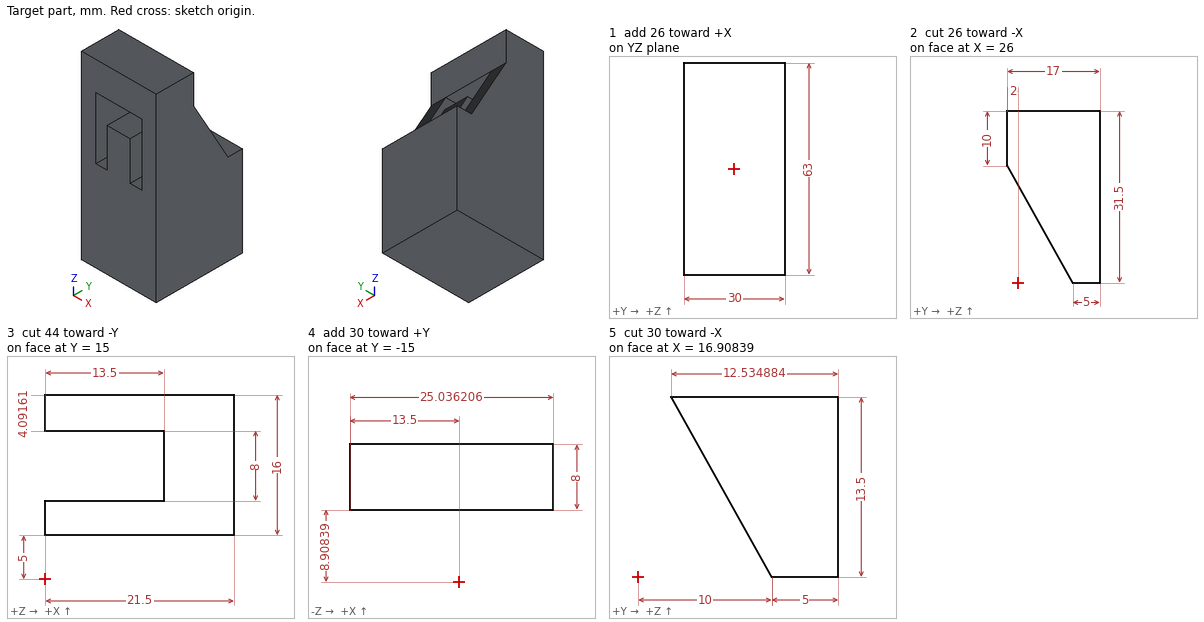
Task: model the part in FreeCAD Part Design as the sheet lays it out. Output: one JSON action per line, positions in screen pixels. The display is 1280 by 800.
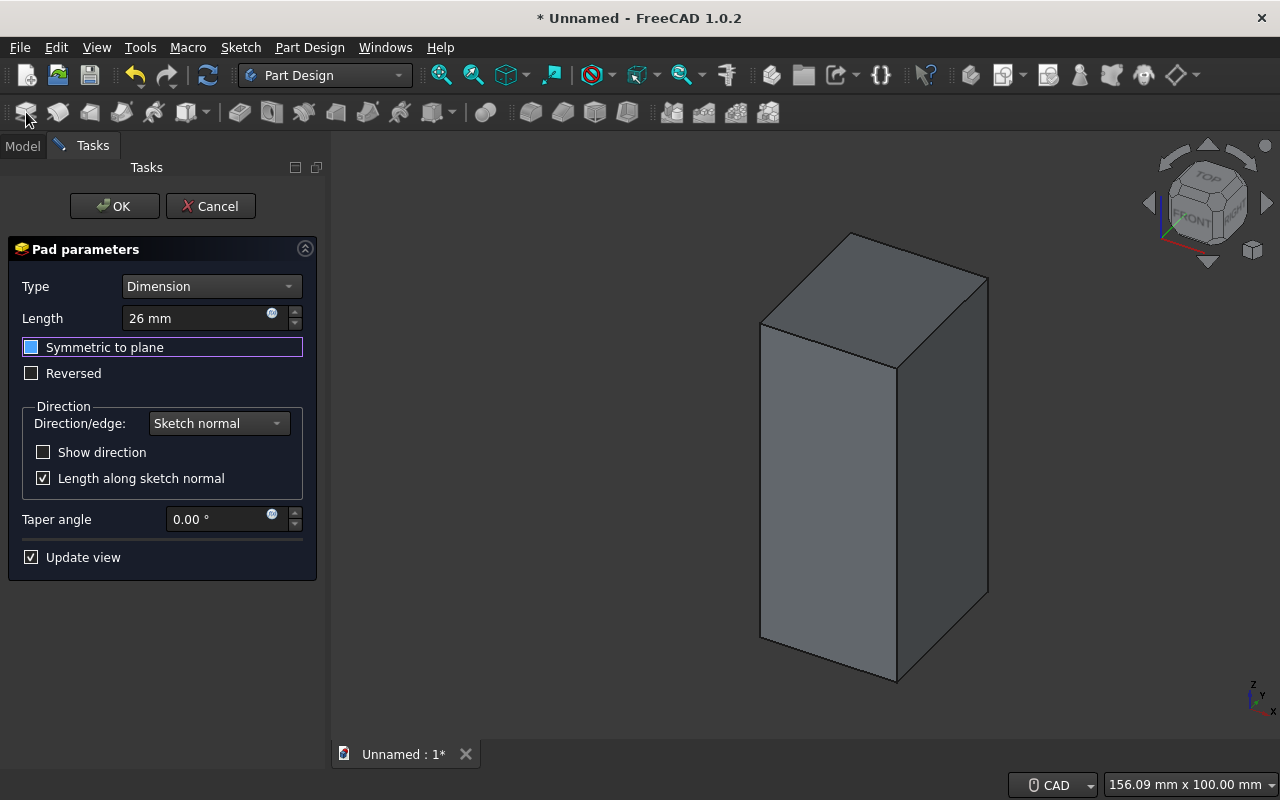
{"action": "left_click", "coordinate": [115, 206]}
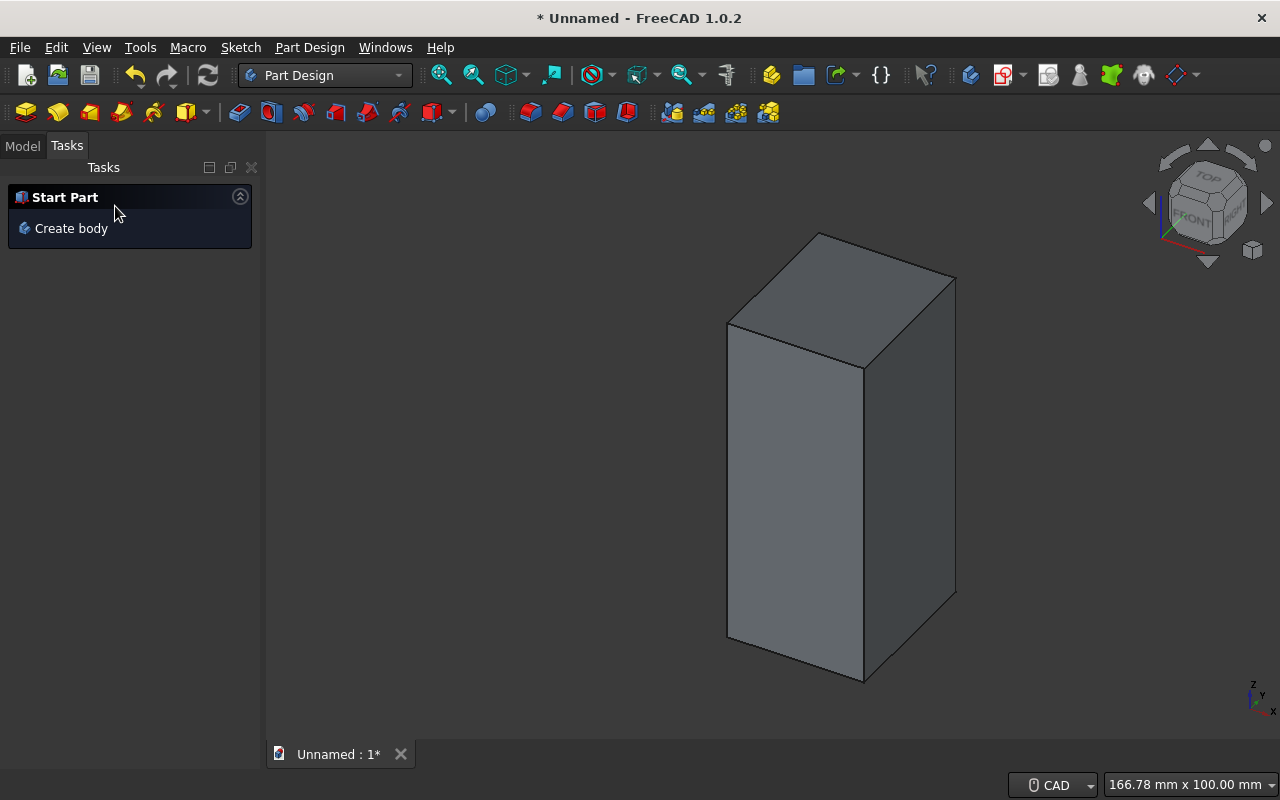
{"action": "left_click", "coordinate": [910, 524]}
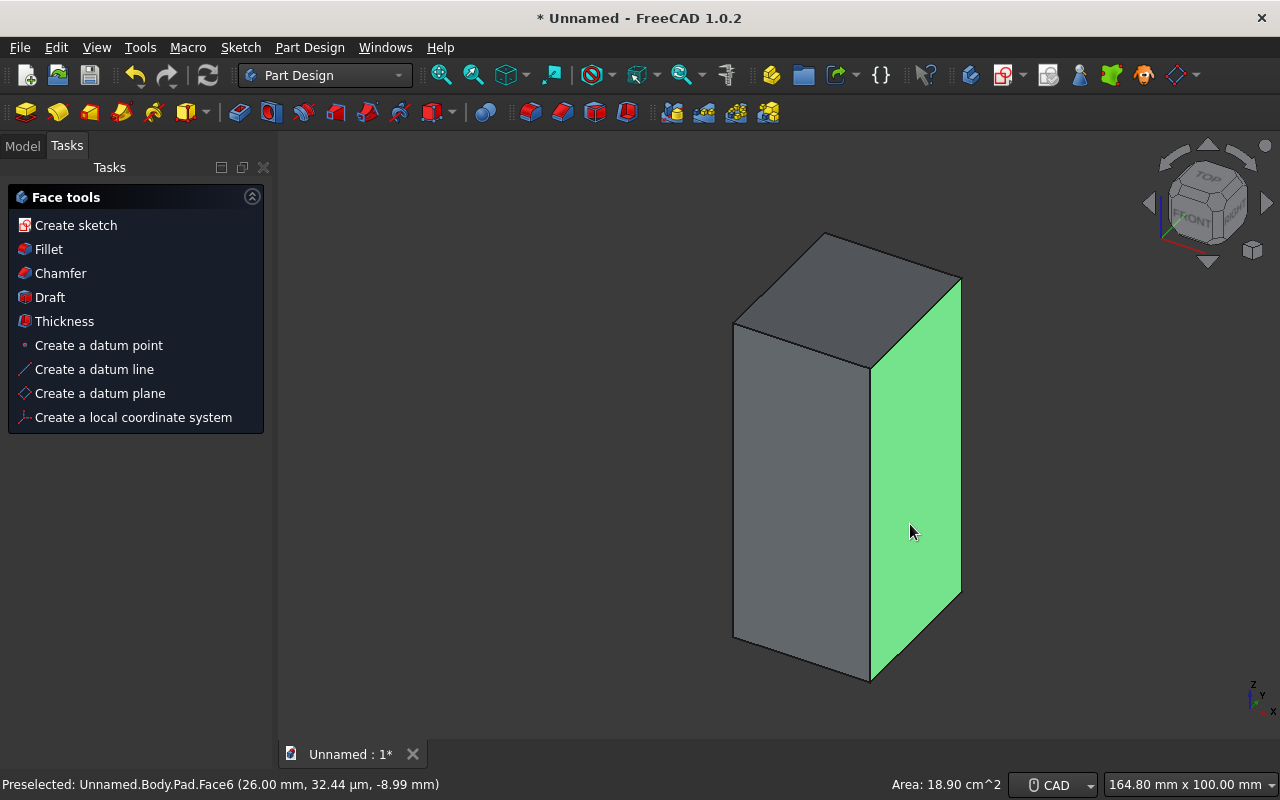
{"action": "left_click", "coordinate": [1004, 76]}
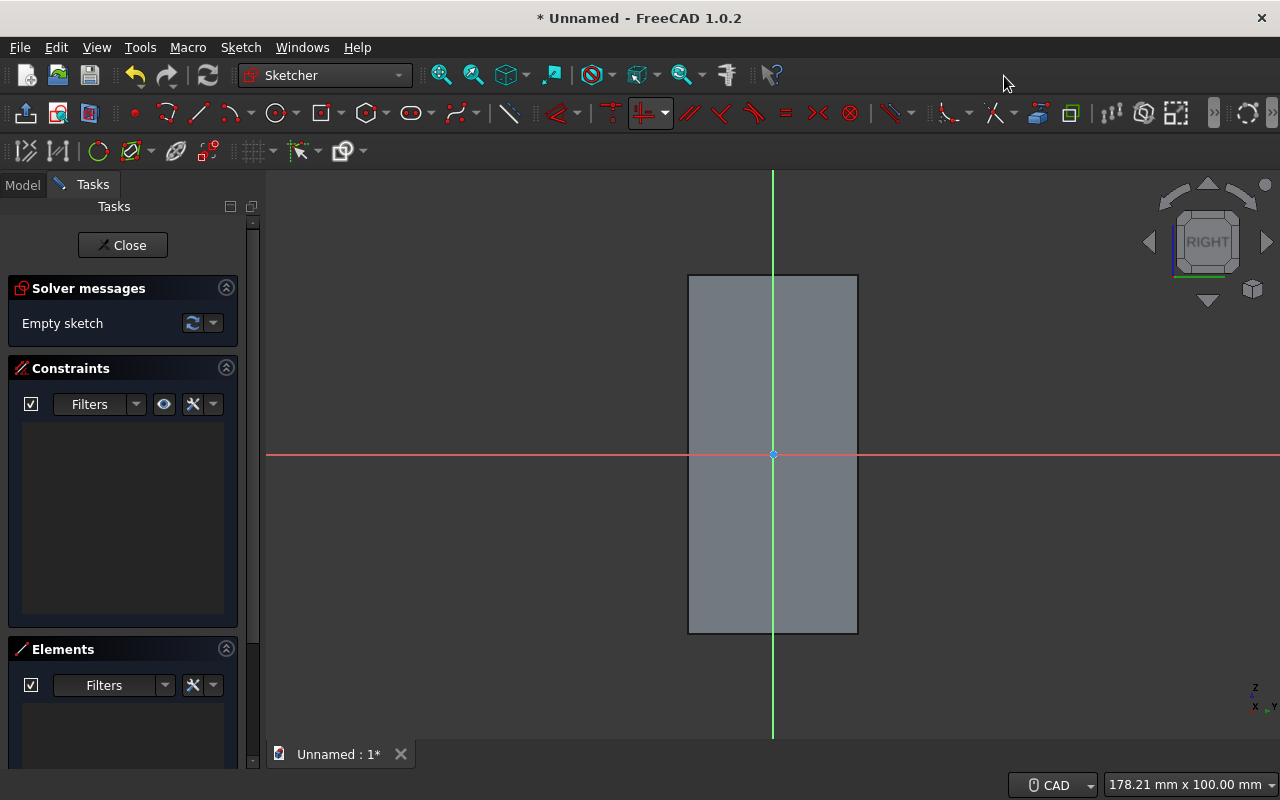
{"action": "scroll", "coordinate": [896, 292], "scroll_direction": "up", "scroll_amount": 4}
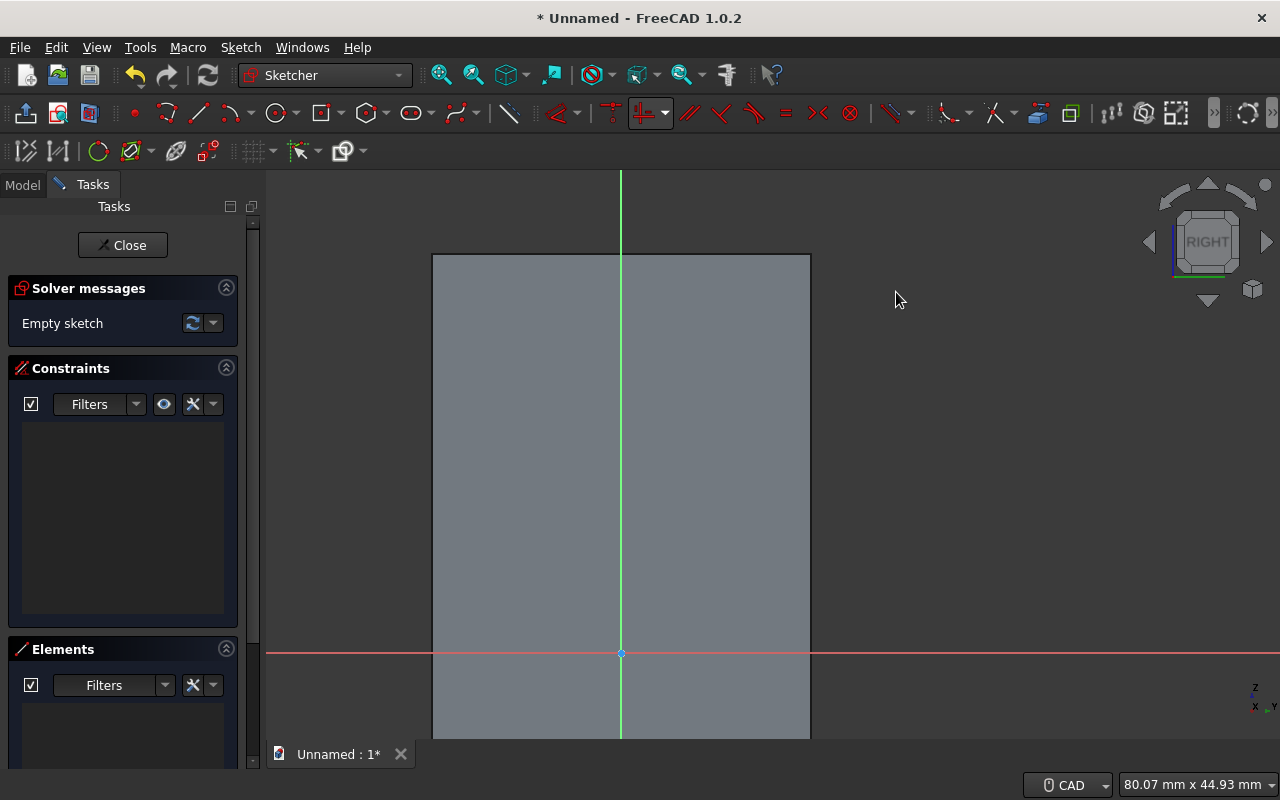
{"action": "key", "text": "g m"}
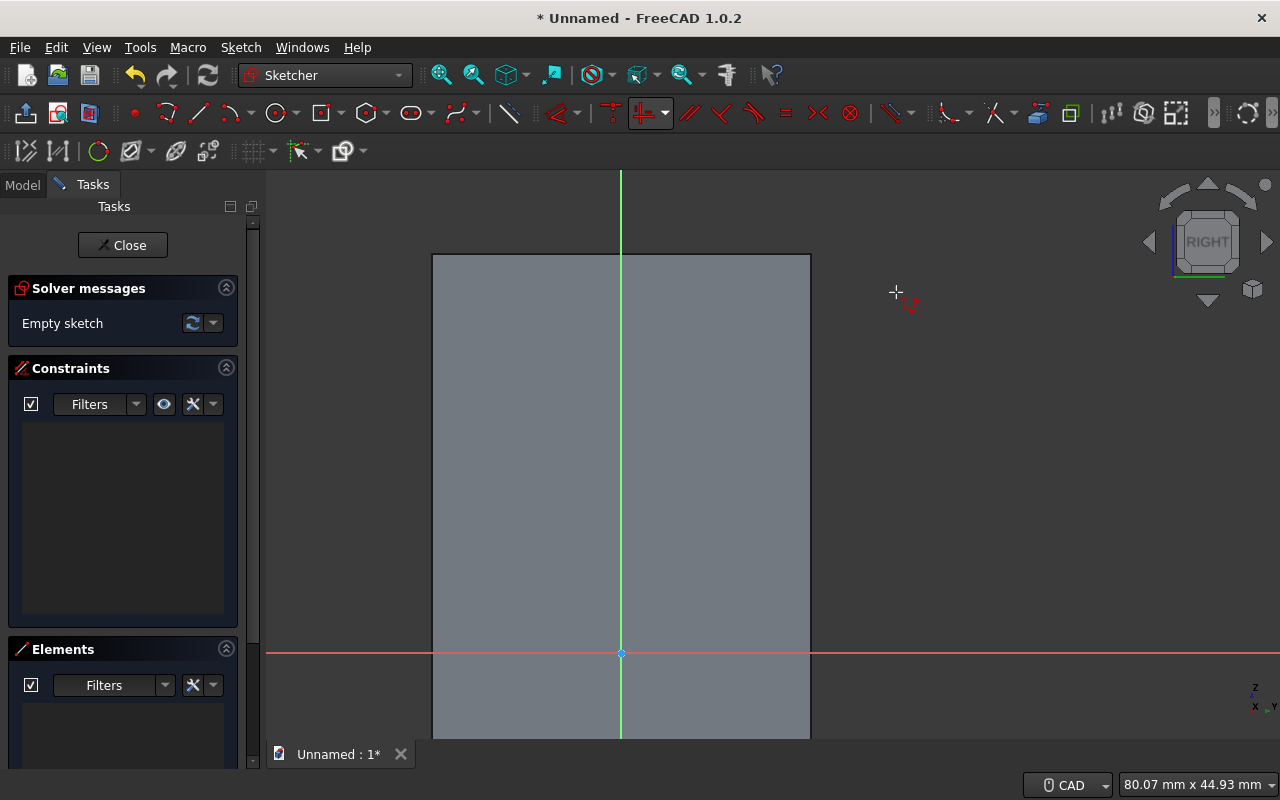
{"action": "left_click", "coordinate": [748, 653]}
{"action": "left_click", "coordinate": [811, 644]}
{"action": "left_click", "coordinate": [811, 254]}
{"action": "left_click", "coordinate": [596, 254]}
{"action": "left_click", "coordinate": [596, 381]}
{"action": "left_click", "coordinate": [748, 653]}
{"action": "key", "text": "Escape"}
{"action": "key", "text": "Escape"}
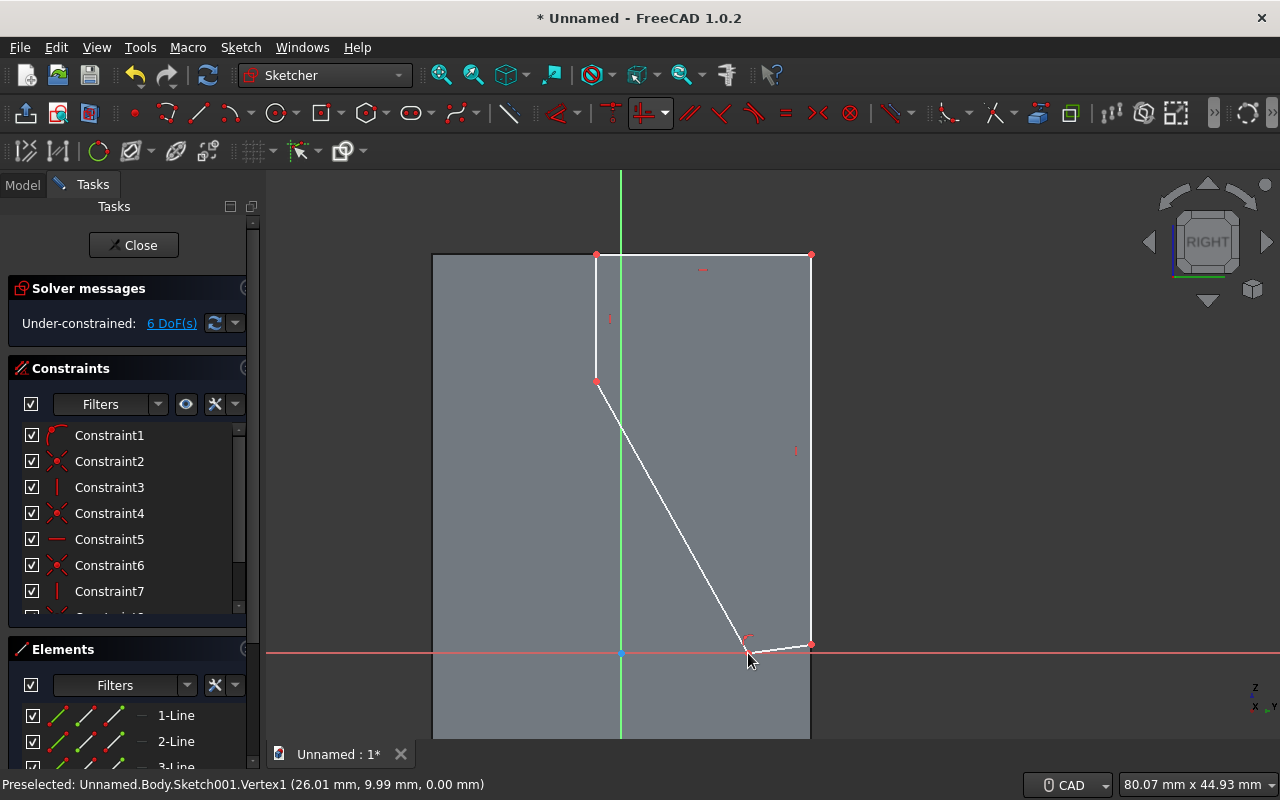
{"action": "left_click", "coordinate": [767, 651]}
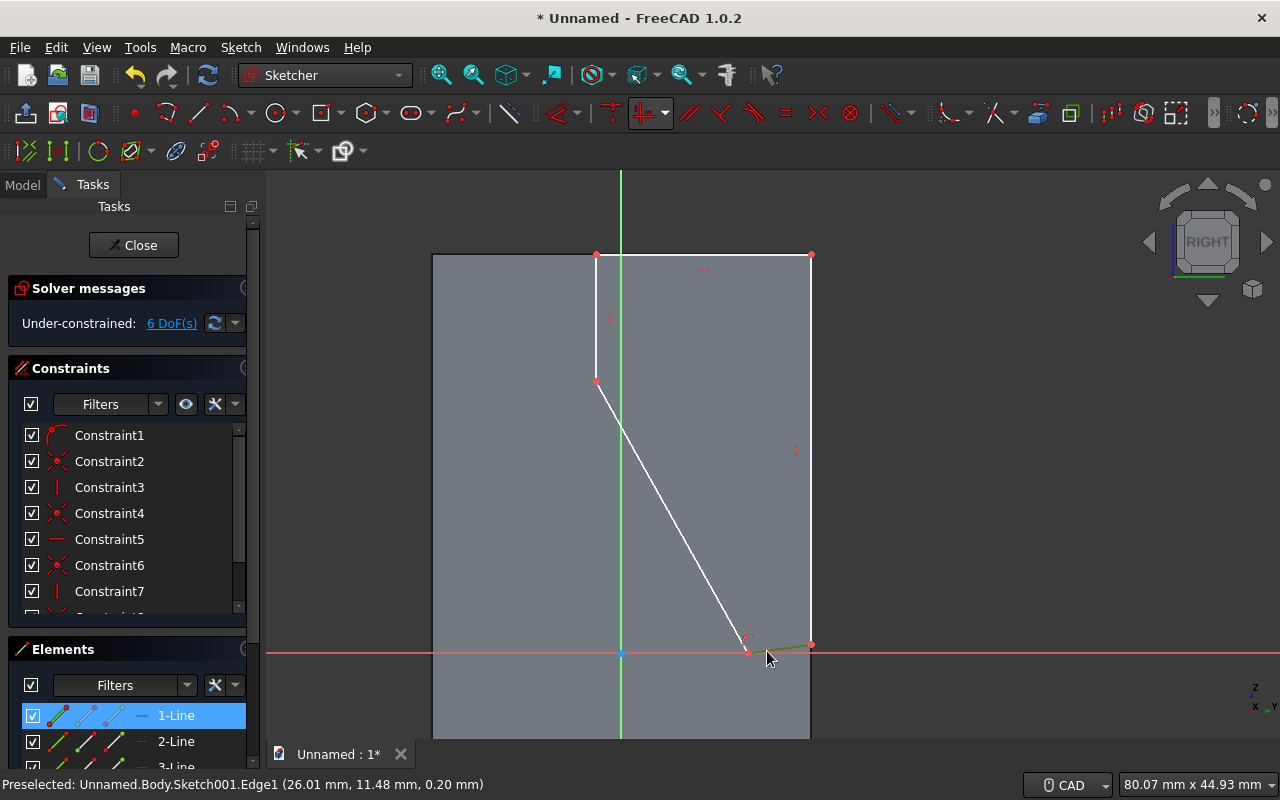
{"action": "key", "text": "h"}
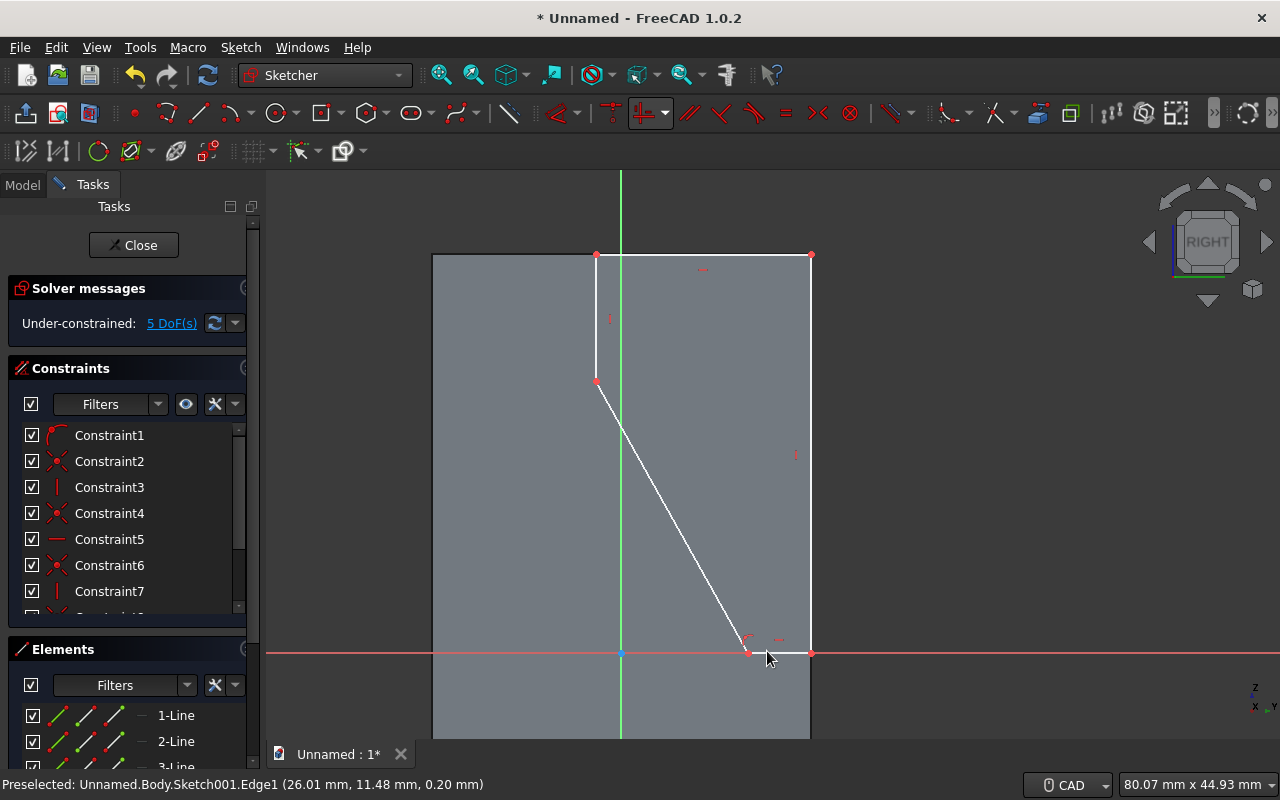
{"action": "key", "text": "d"}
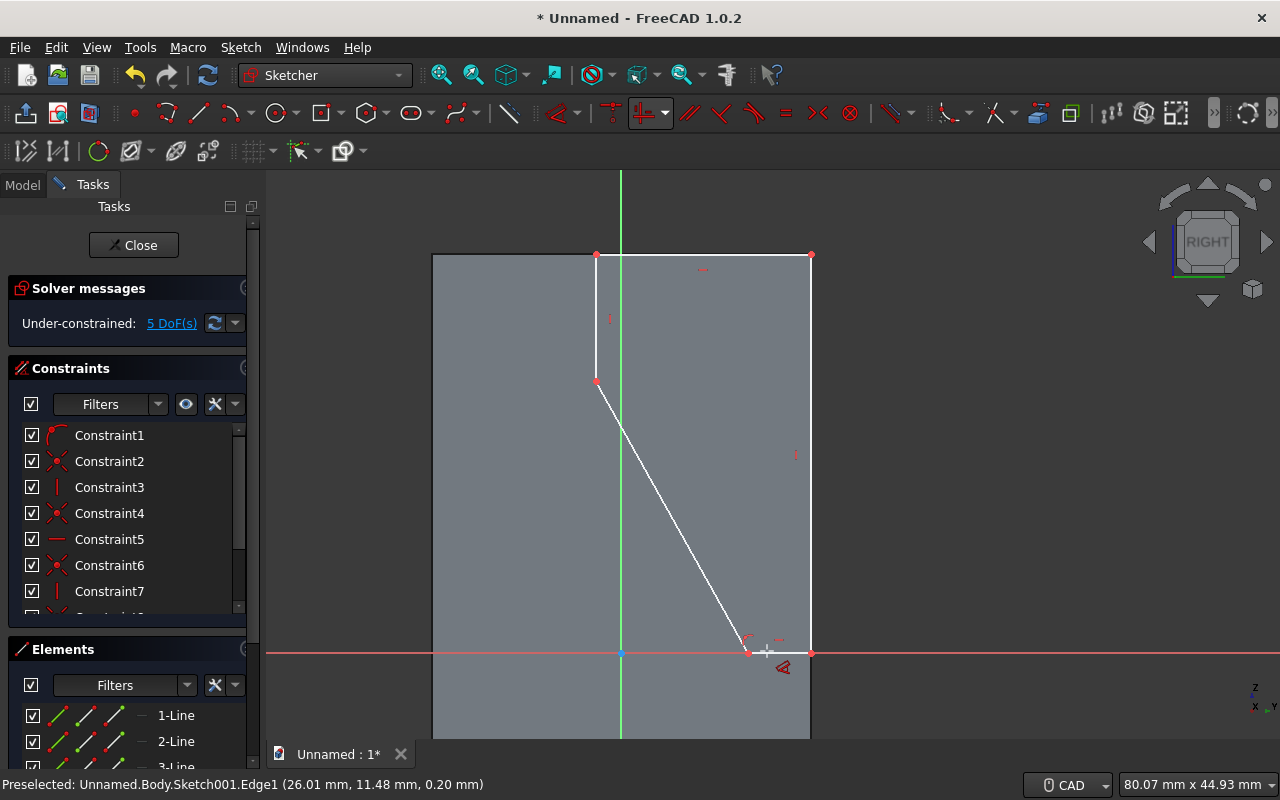
{"action": "left_click", "coordinate": [767, 653]}
{"action": "left_click", "coordinate": [780, 687]}